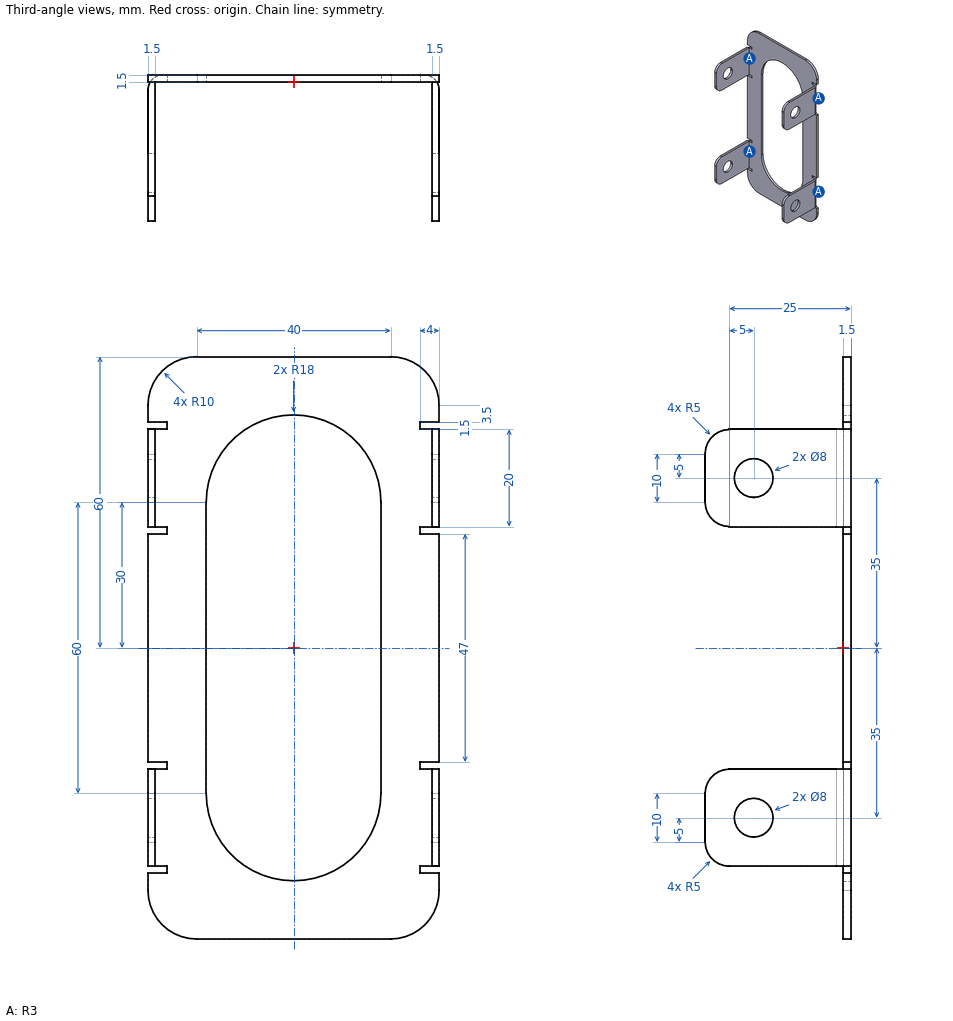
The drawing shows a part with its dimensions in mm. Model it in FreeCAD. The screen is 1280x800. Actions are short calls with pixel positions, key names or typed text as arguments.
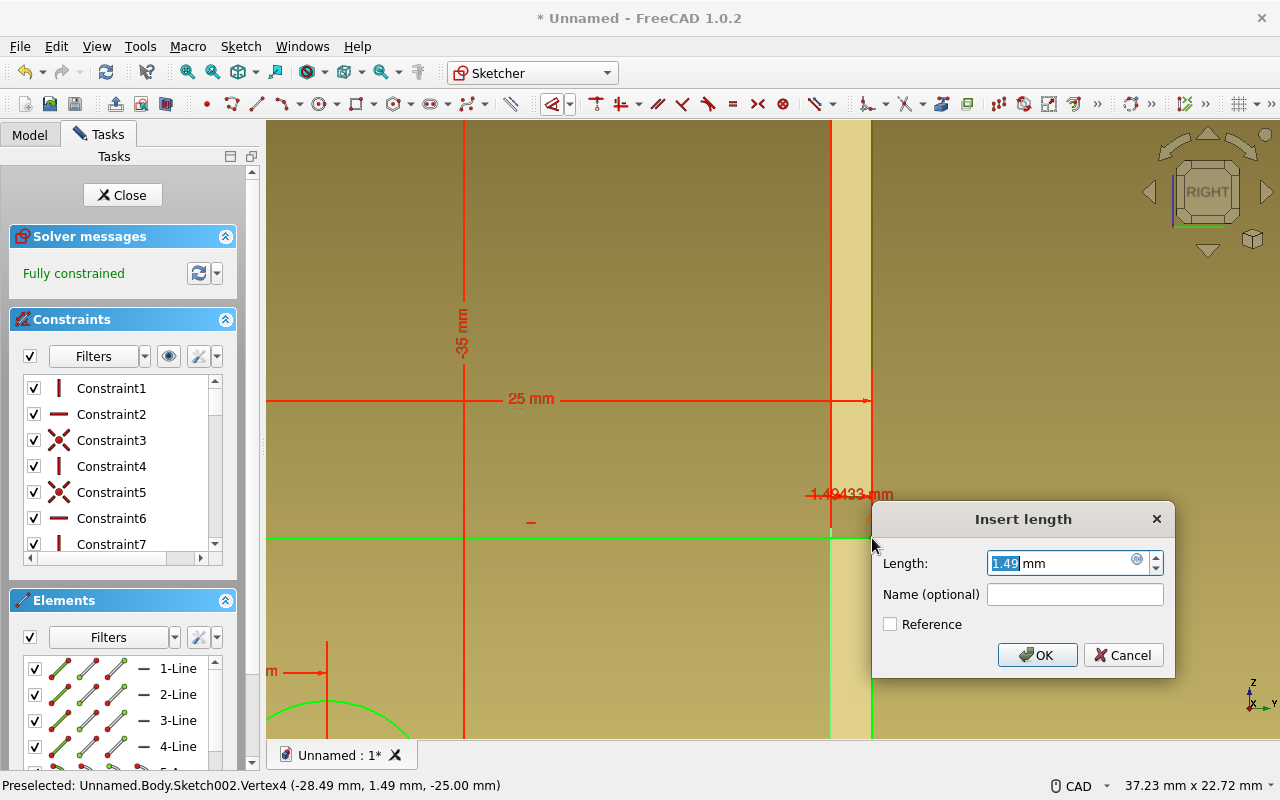
text(1.5)
key(Return)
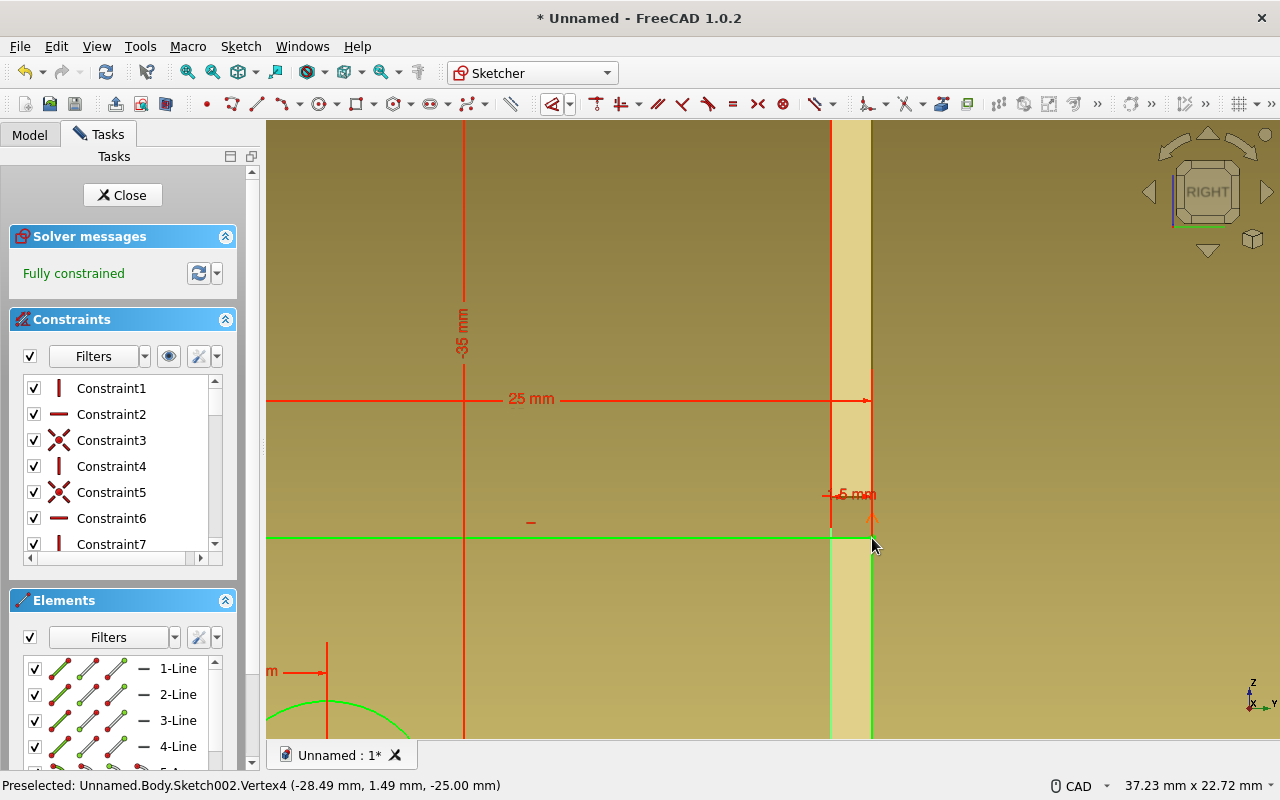
click(123, 195)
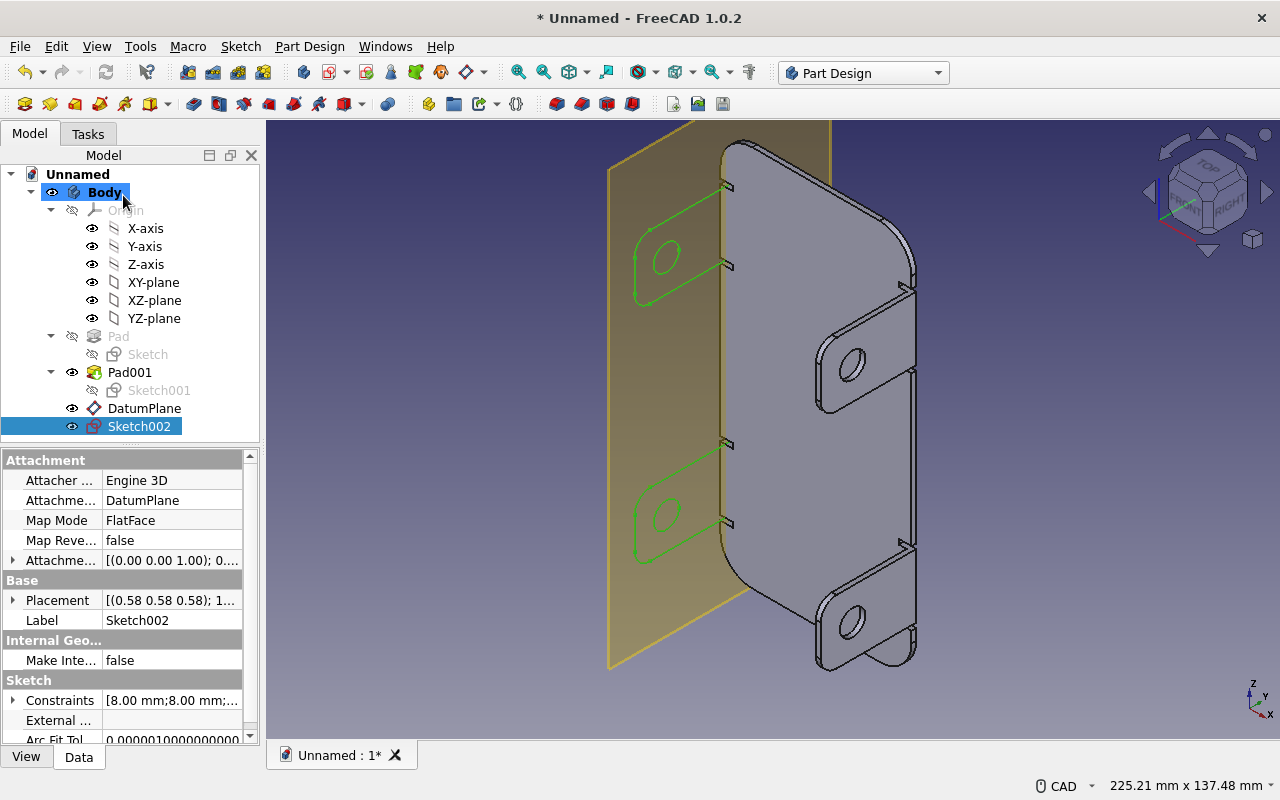
click(25, 104)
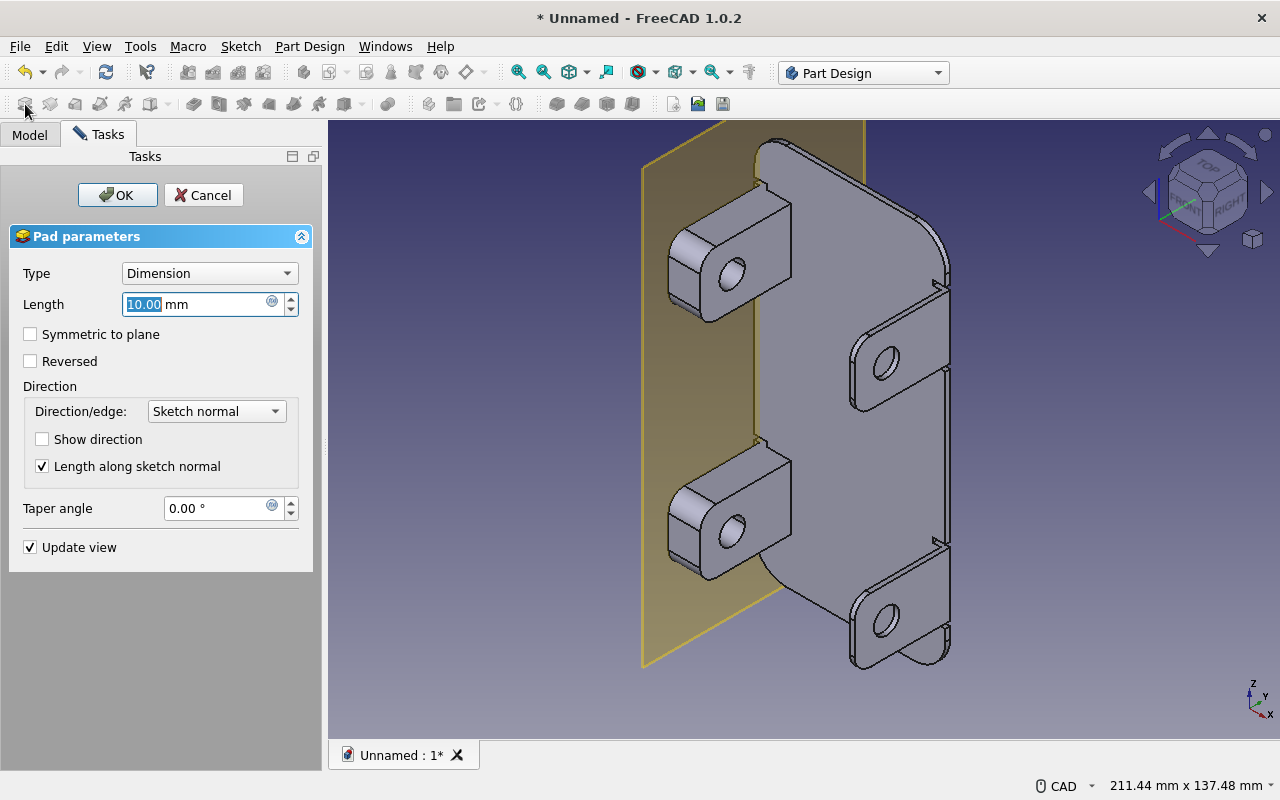
text(1.5)
key(Tab)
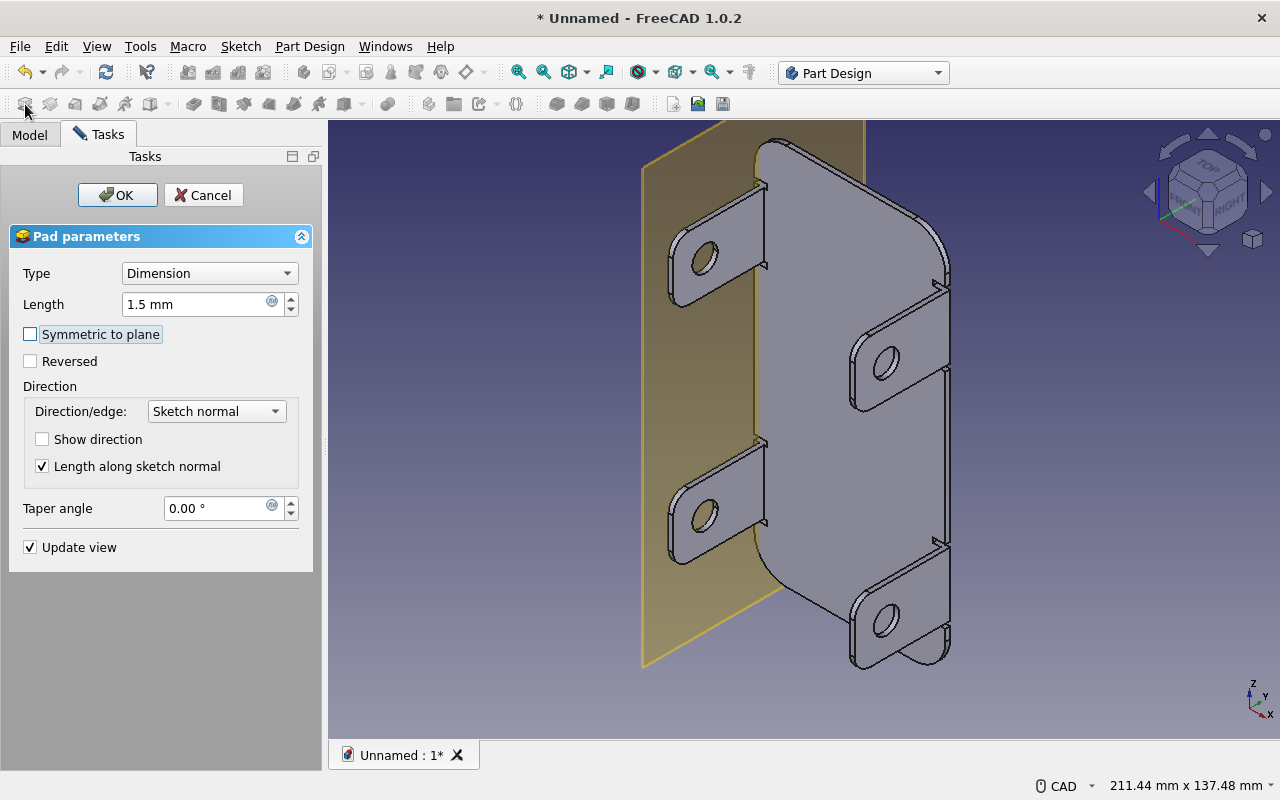
click(31, 361)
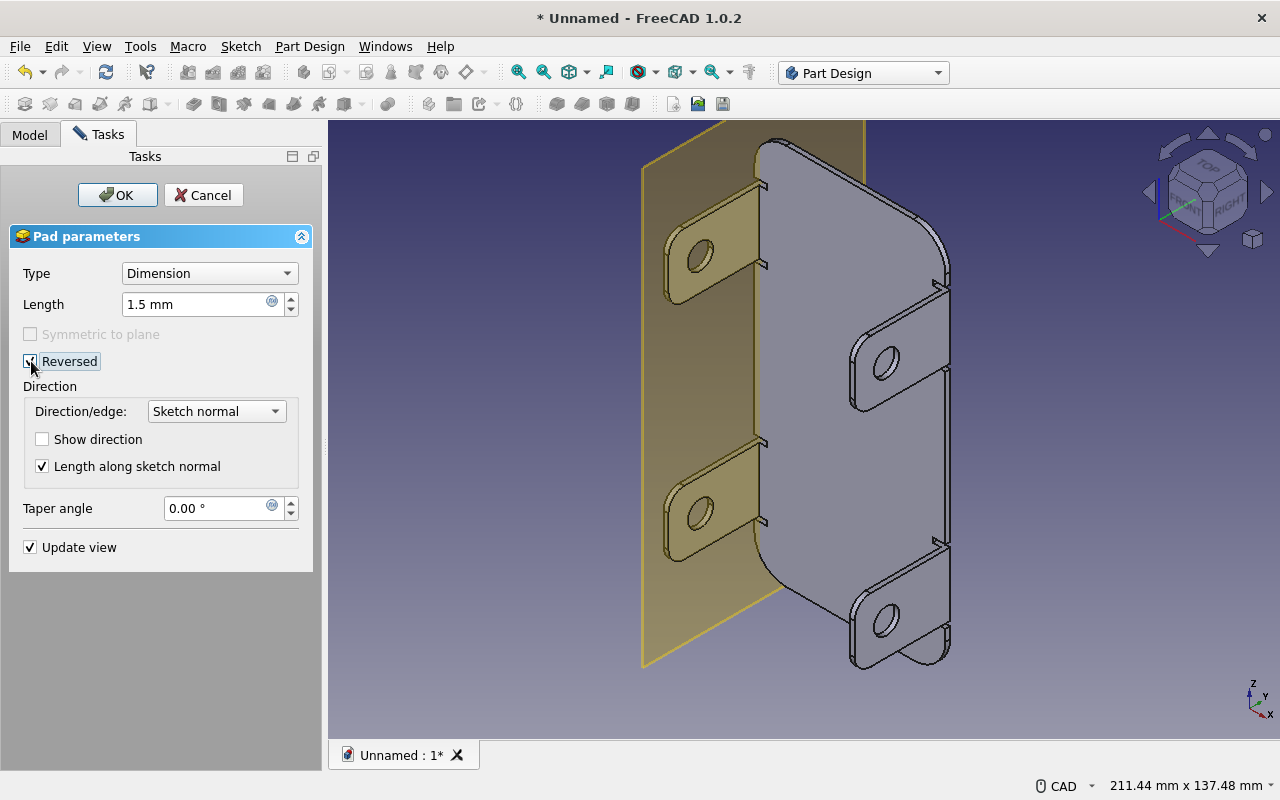
click(118, 195)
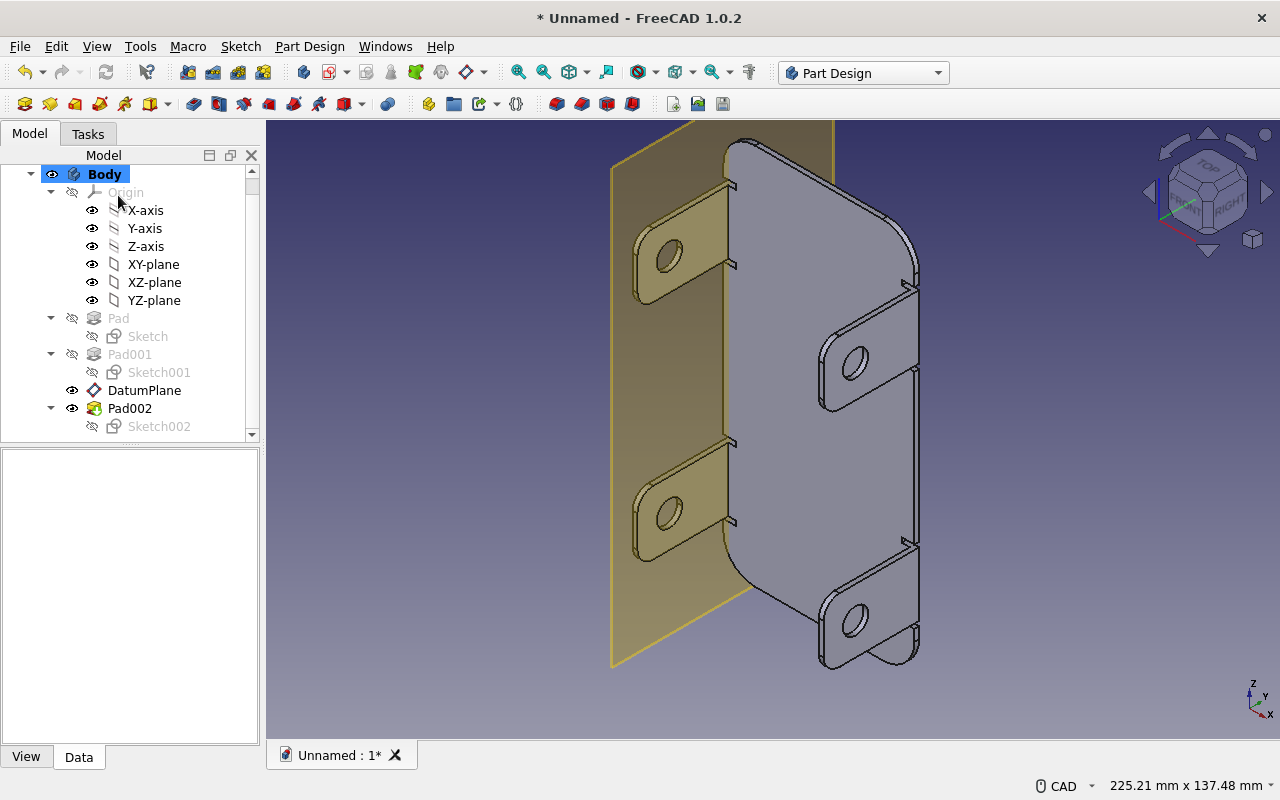
click(117, 390)
key(space)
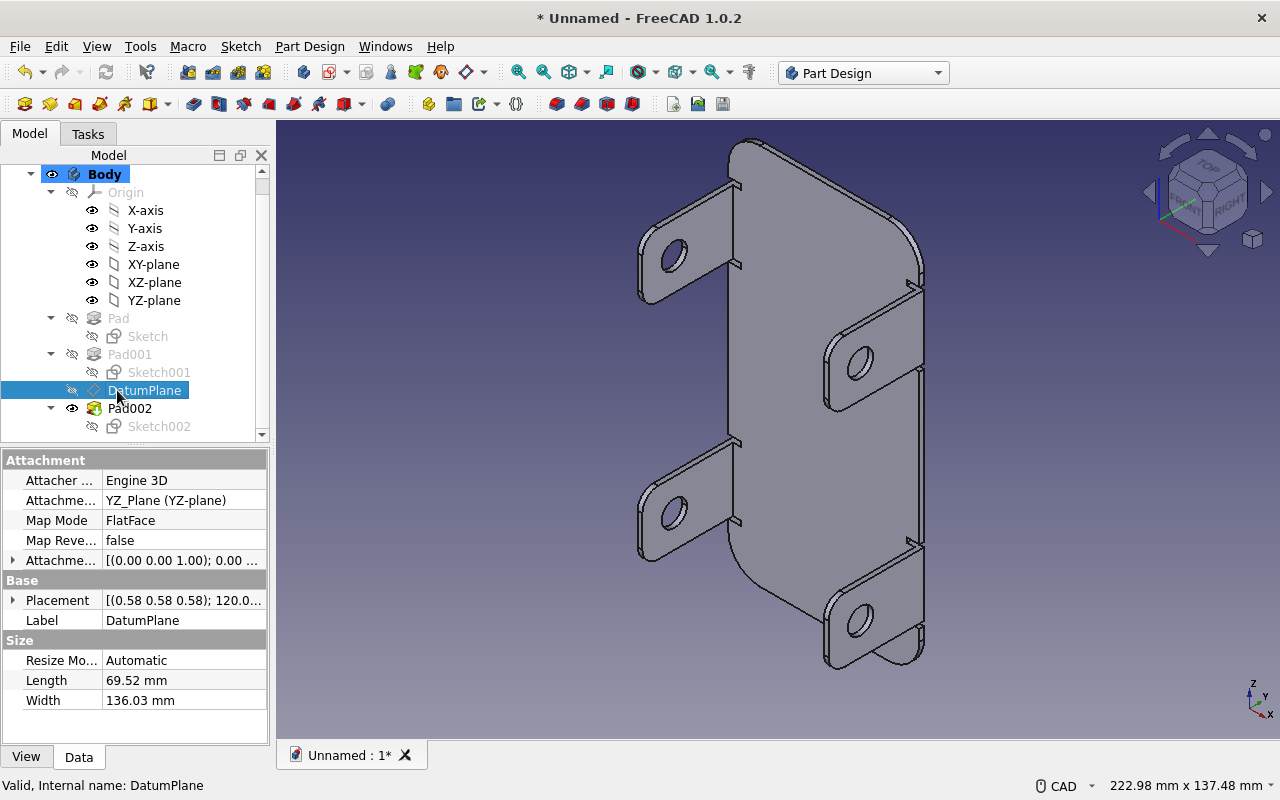
key(2)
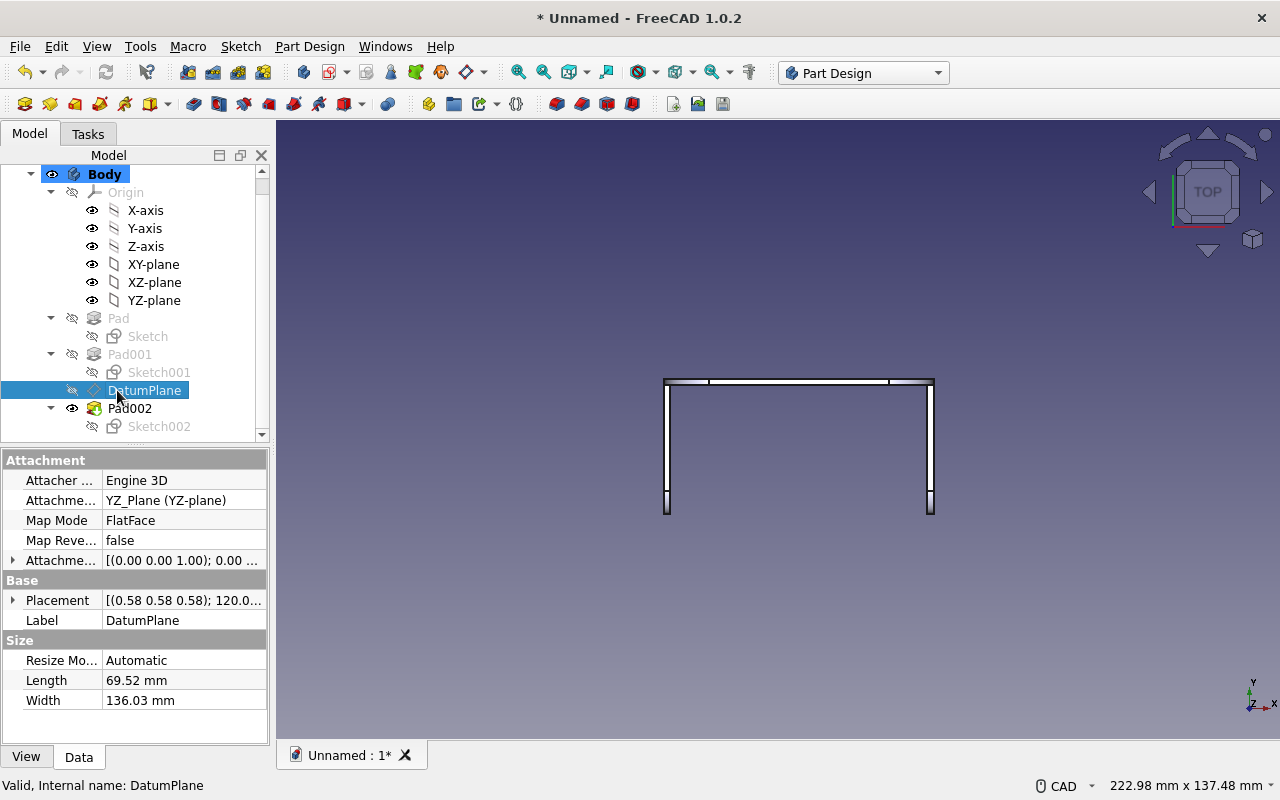
click(519, 72)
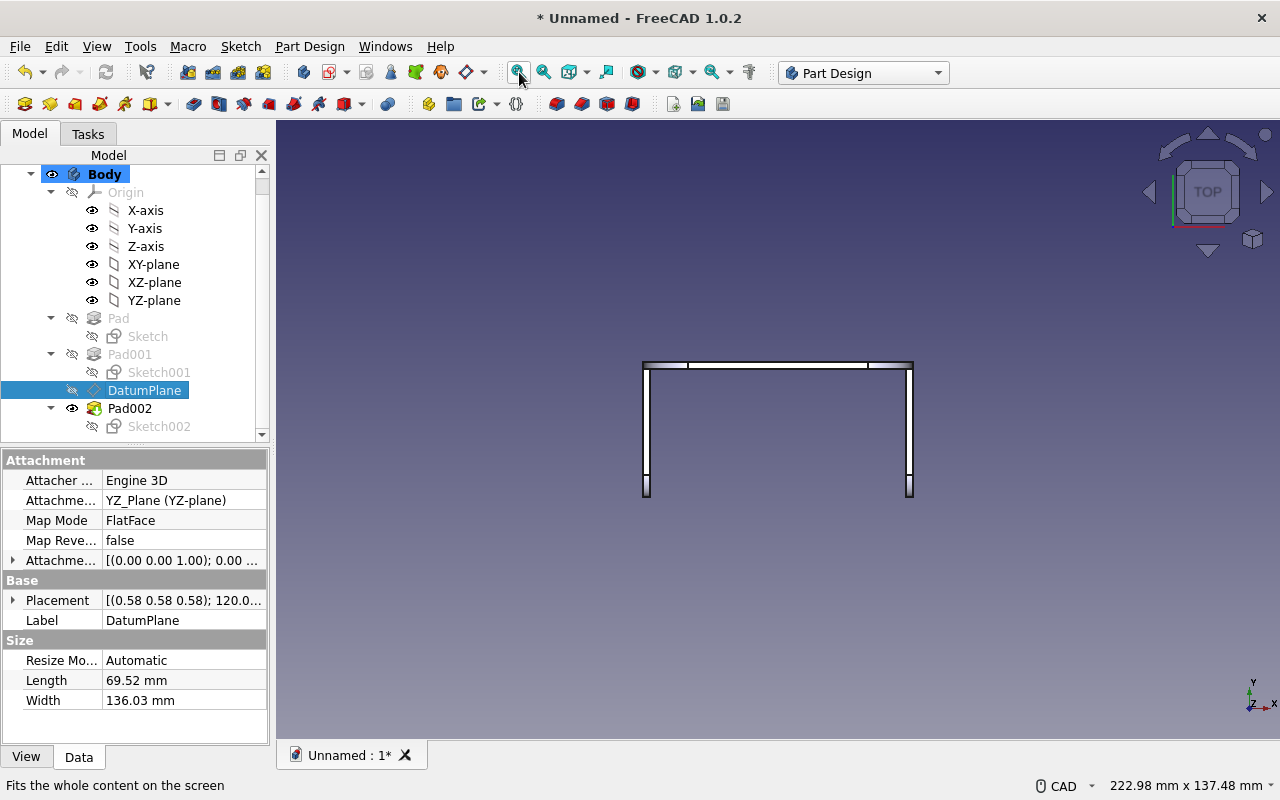
key(0)